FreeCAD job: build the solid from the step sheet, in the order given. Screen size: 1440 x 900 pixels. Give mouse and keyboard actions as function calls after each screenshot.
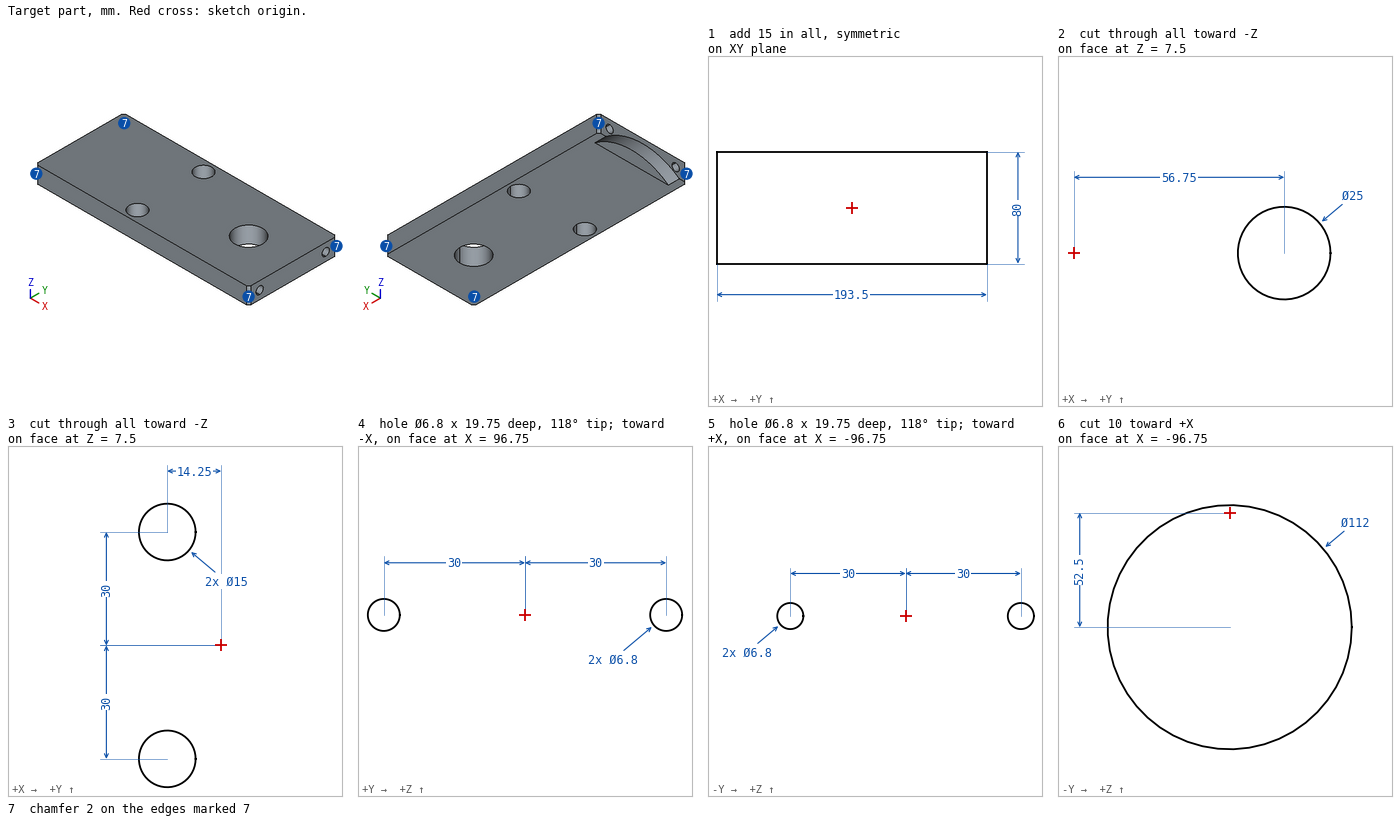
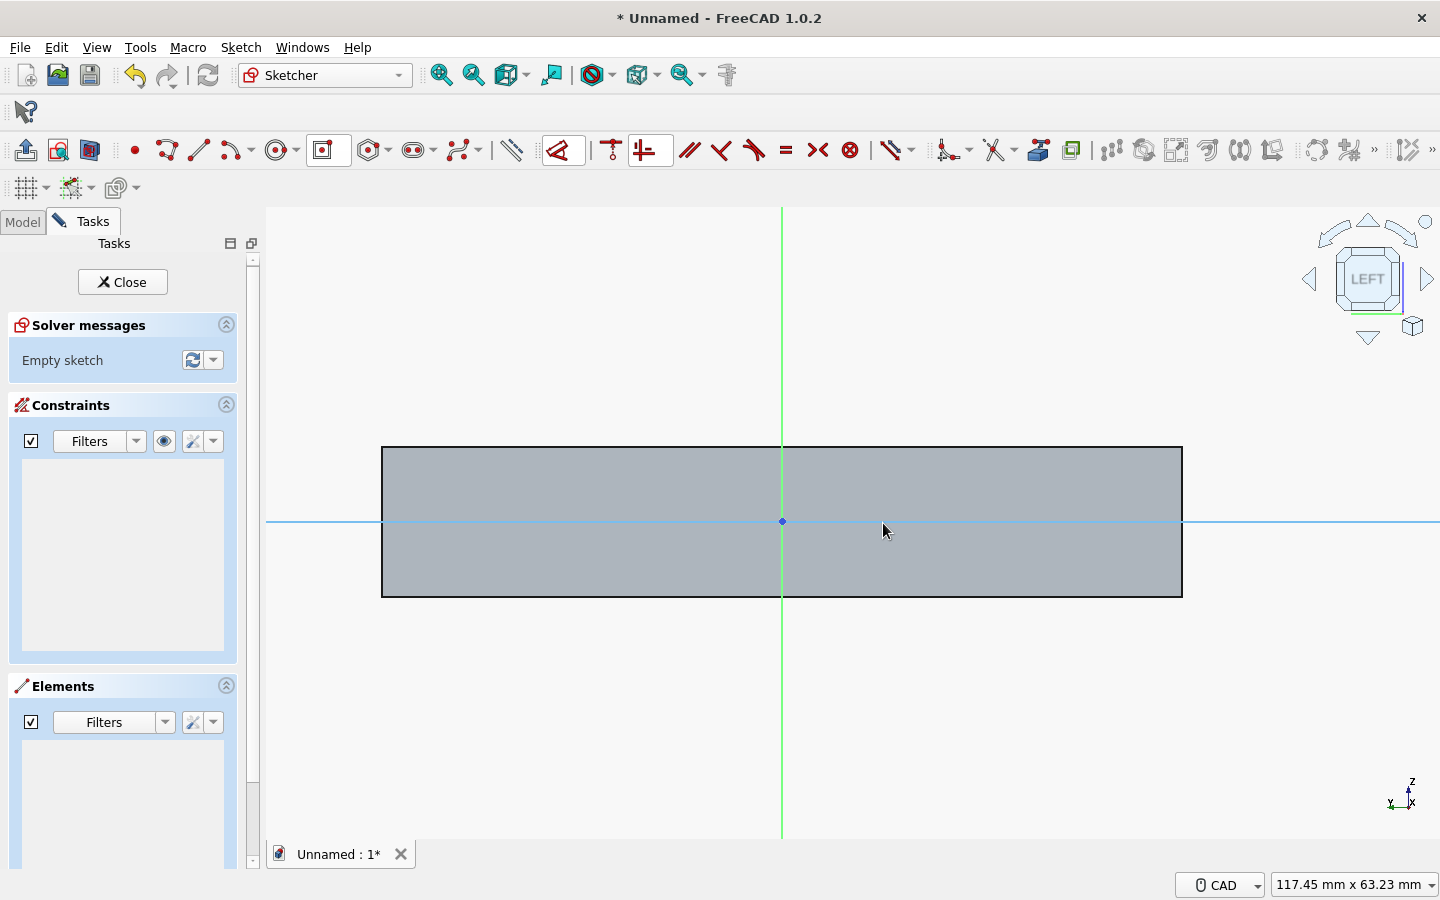
click(276, 150)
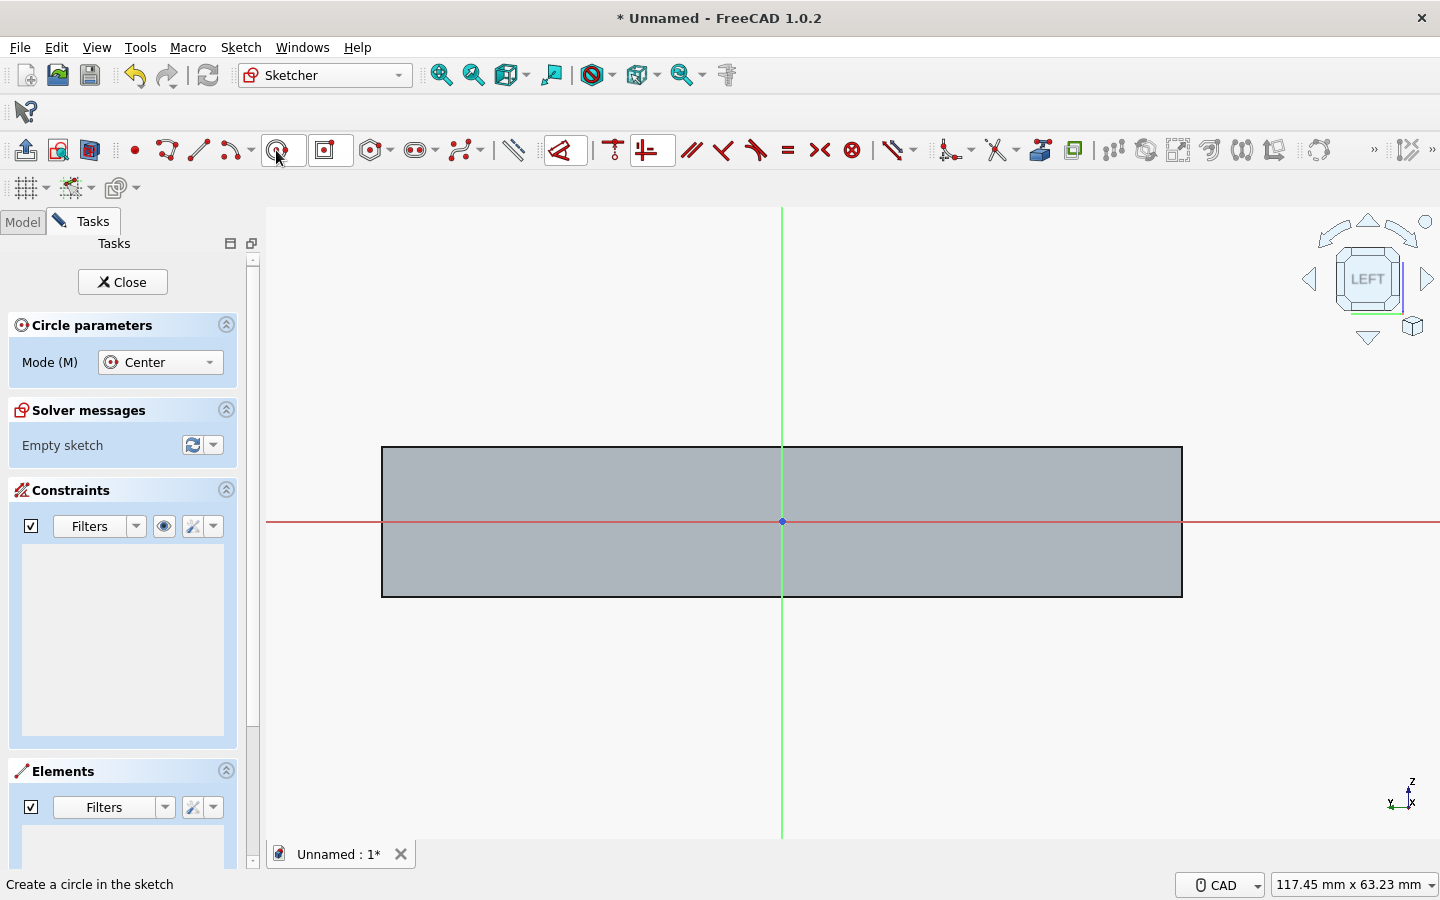
click(482, 522)
move(506, 498)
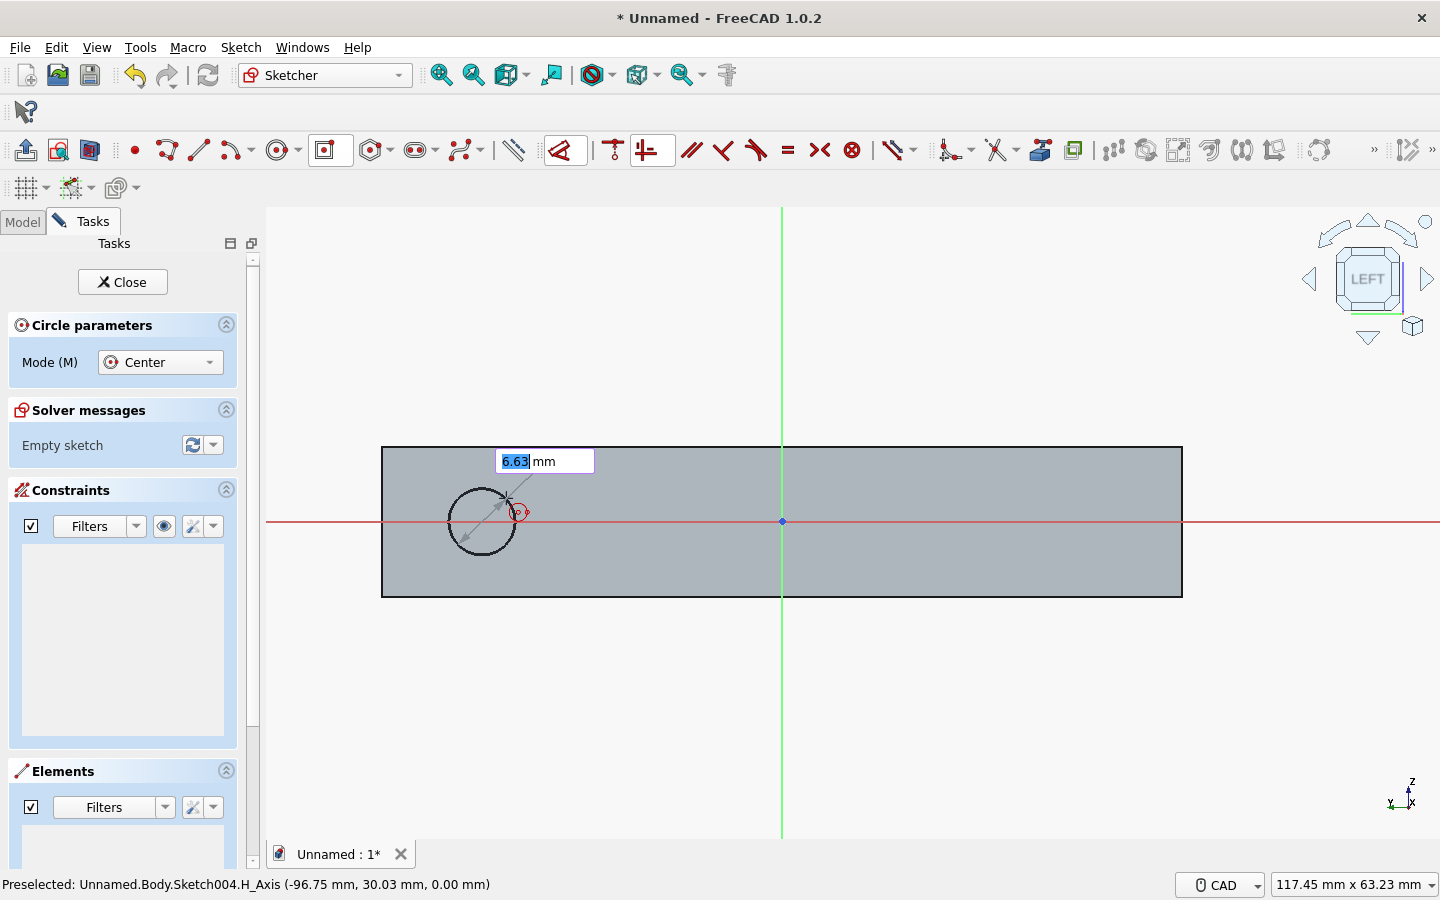
text(6.8)
key(Return)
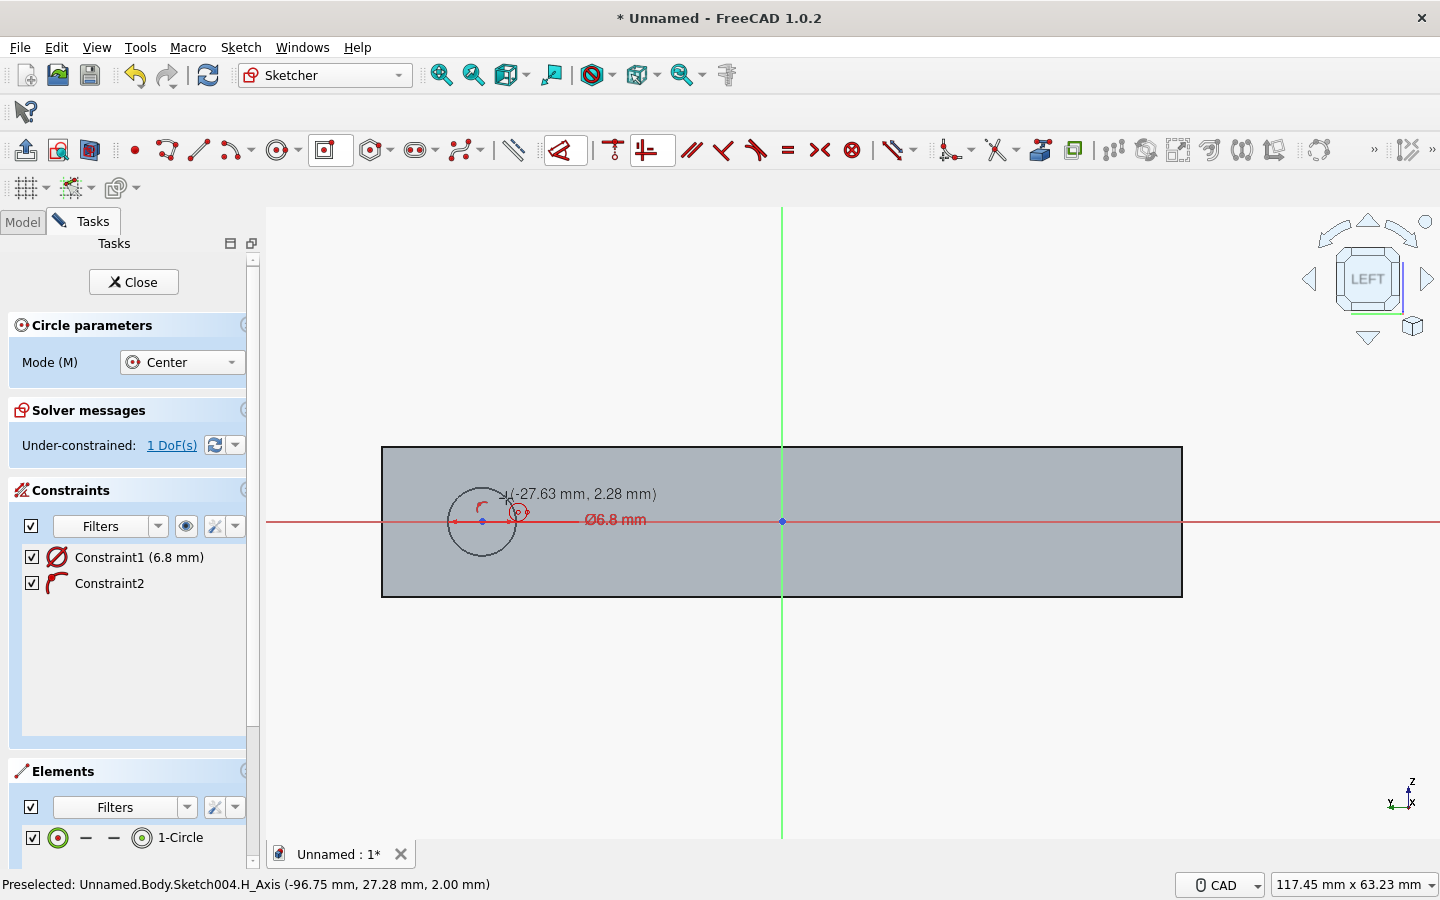
click(1082, 522)
move(1106, 498)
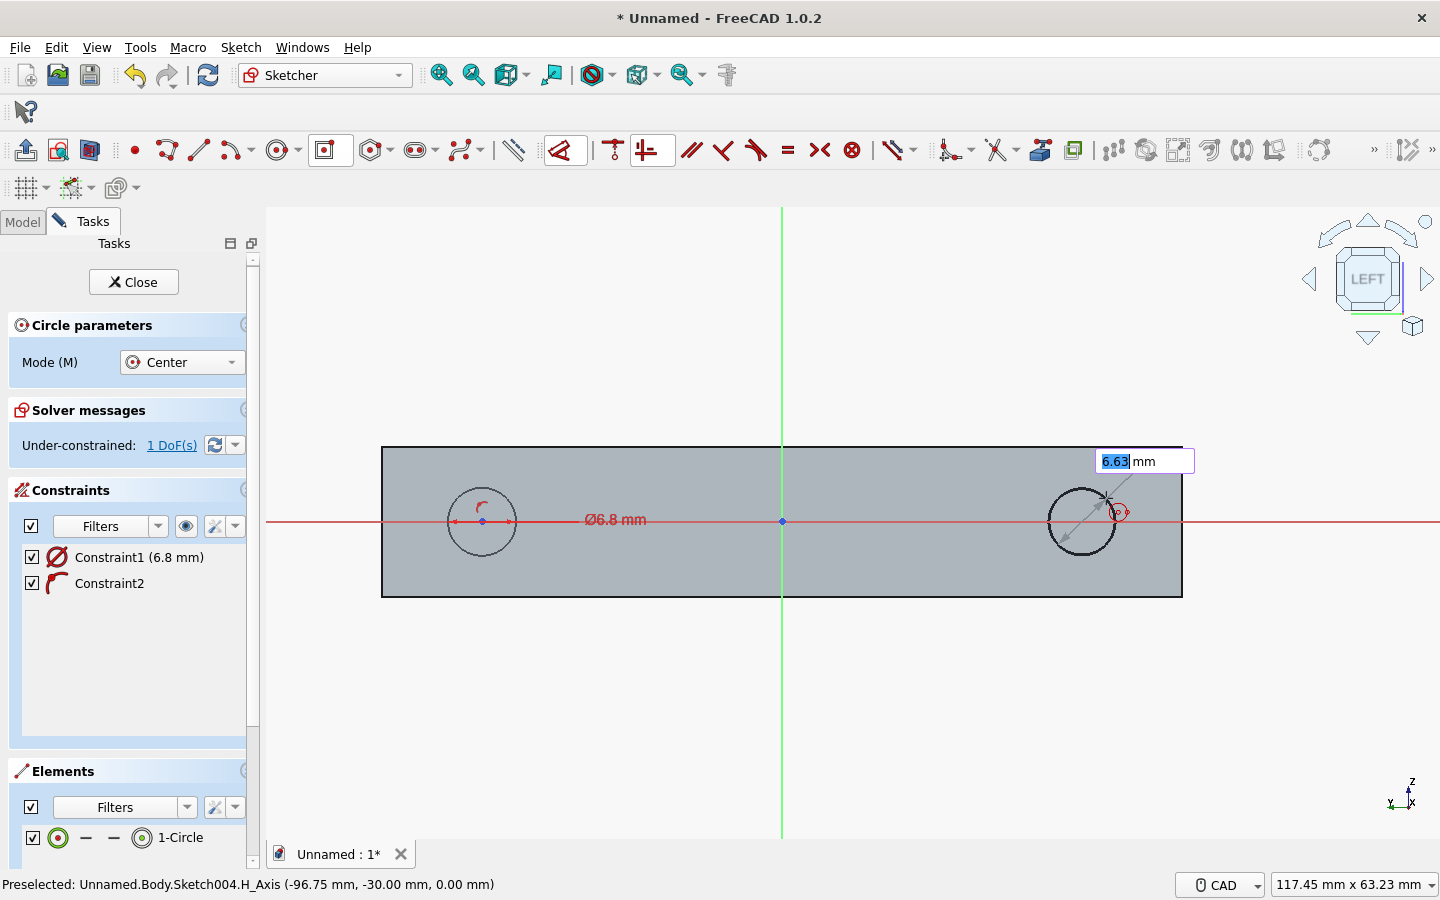
text(6.8)
key(Return)
key(Escape)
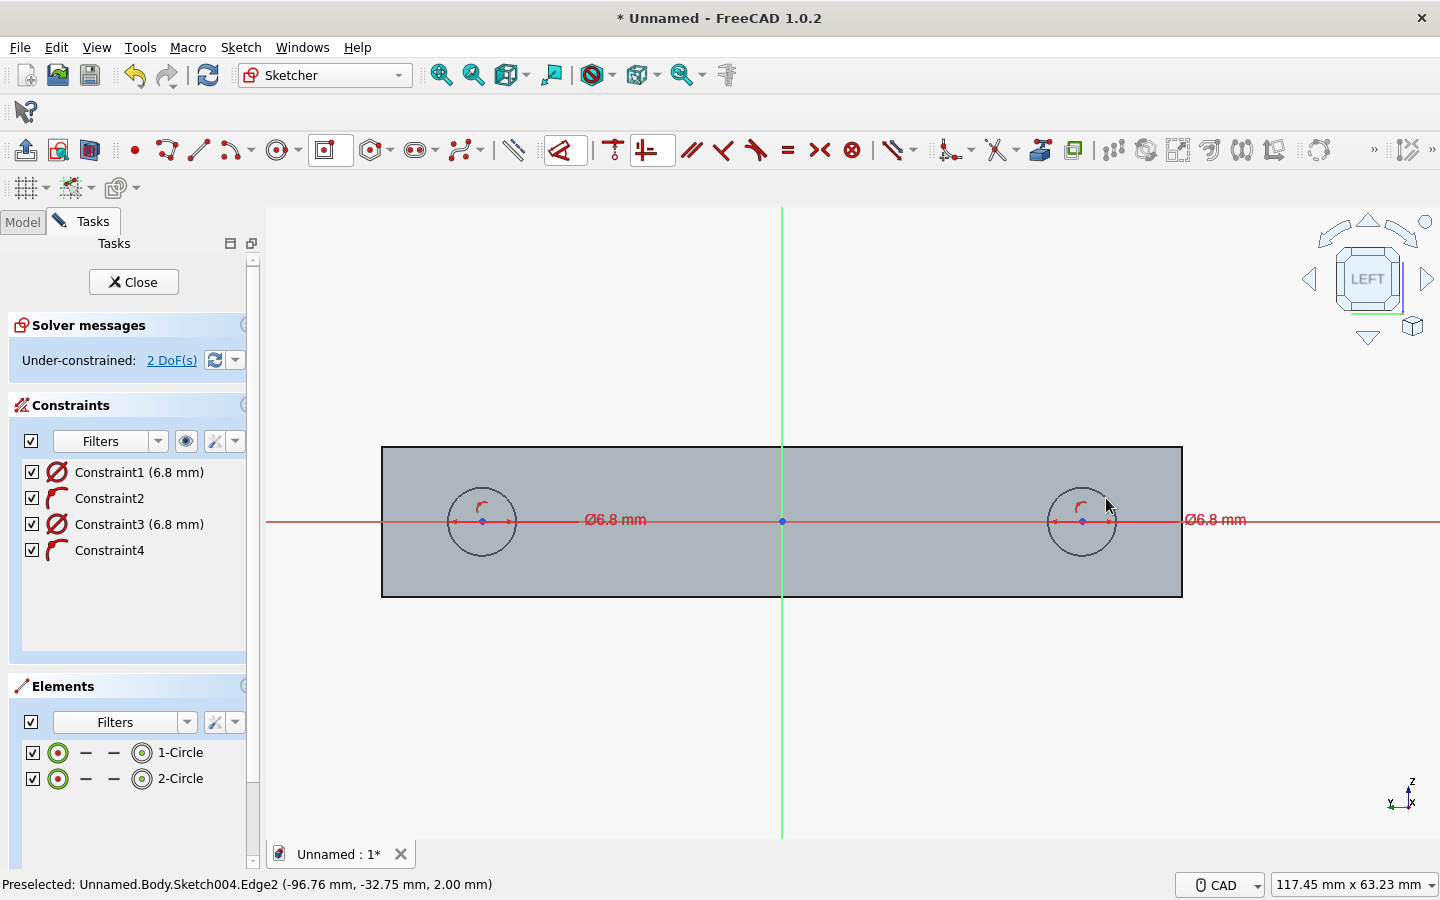
click(482, 522)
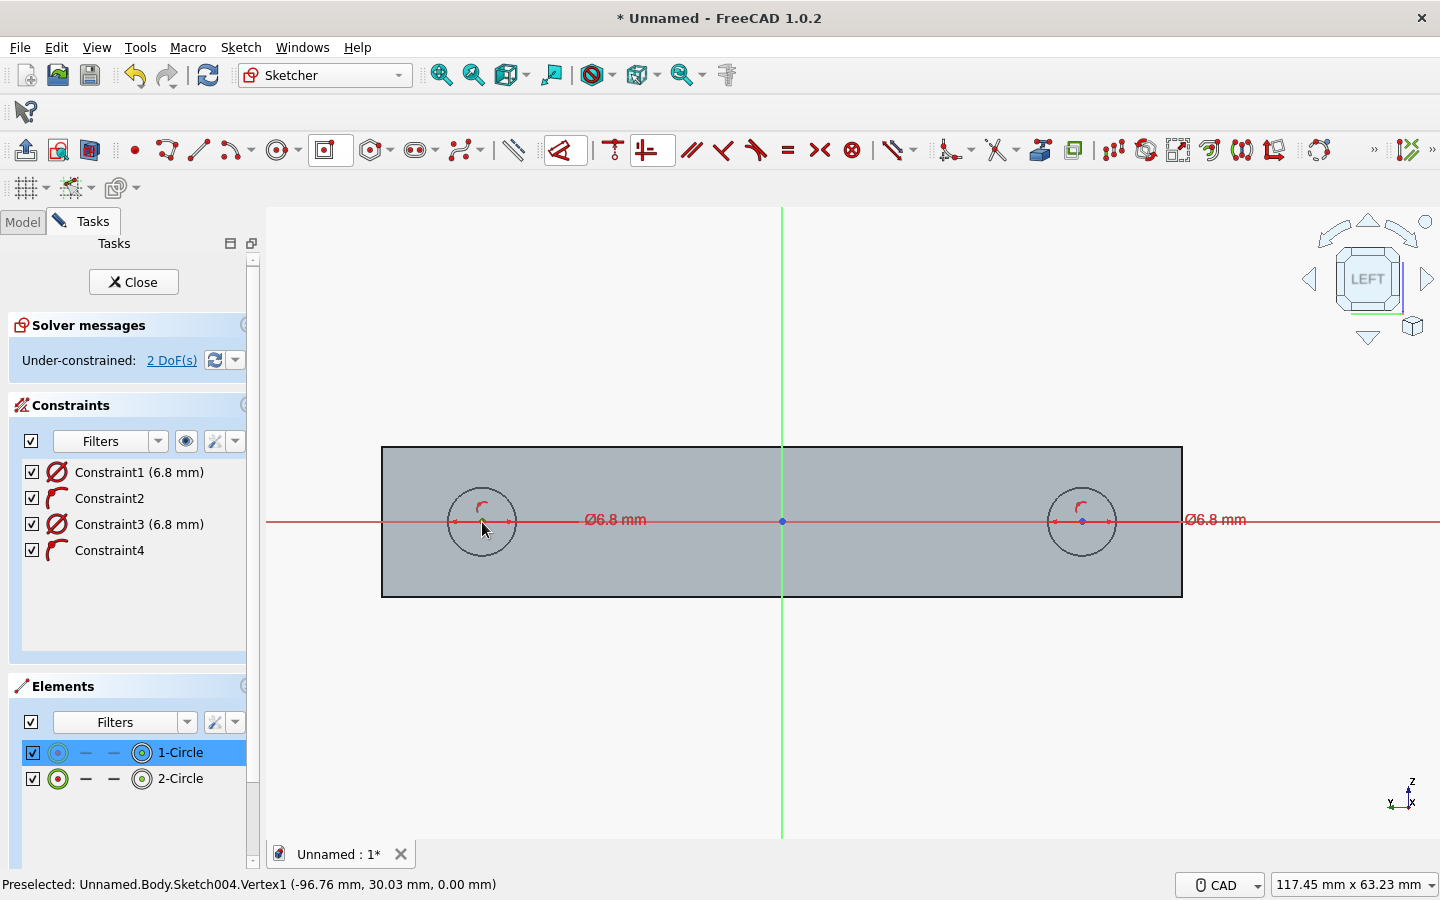
click(582, 150)